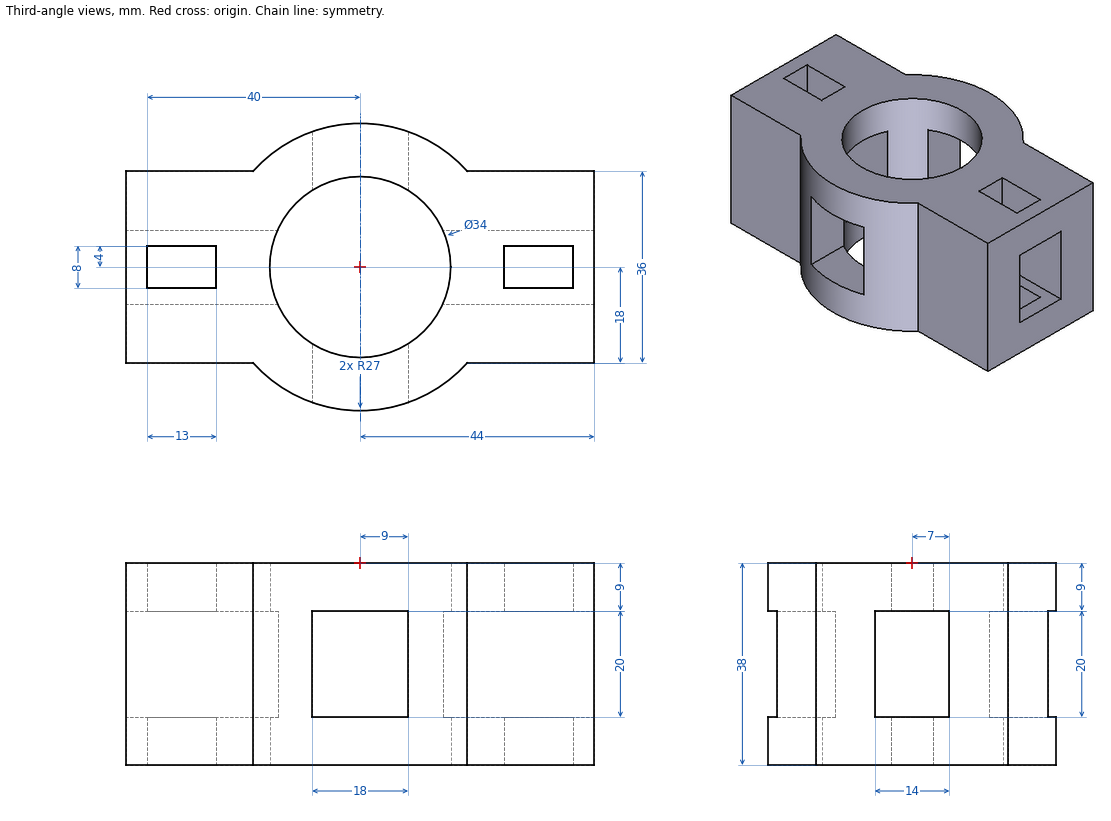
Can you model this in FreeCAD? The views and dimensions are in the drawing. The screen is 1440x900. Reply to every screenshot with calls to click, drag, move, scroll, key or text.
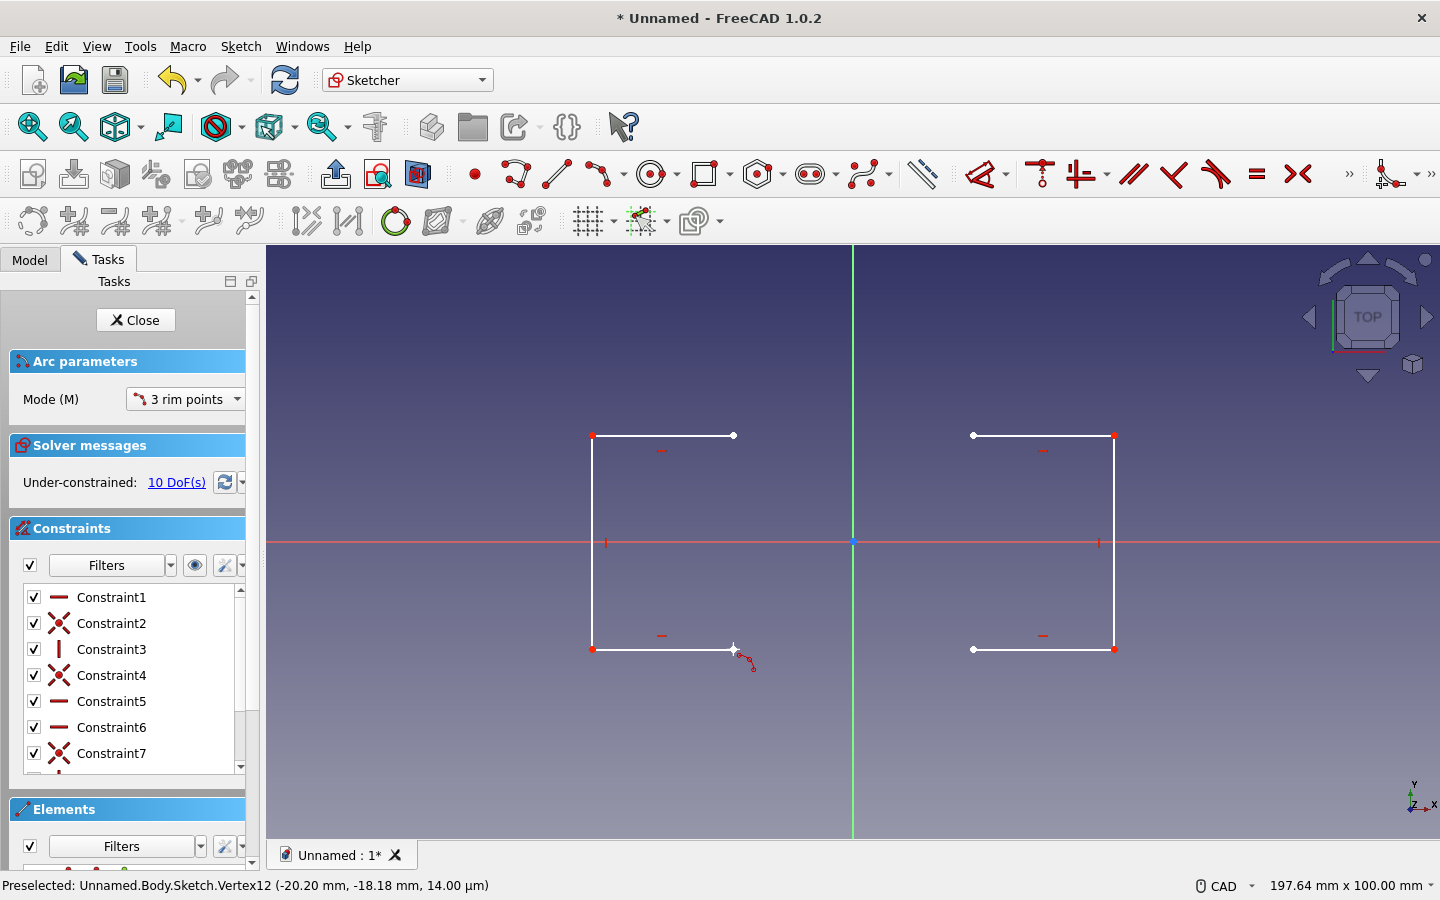
click(973, 436)
click(733, 436)
click(880, 384)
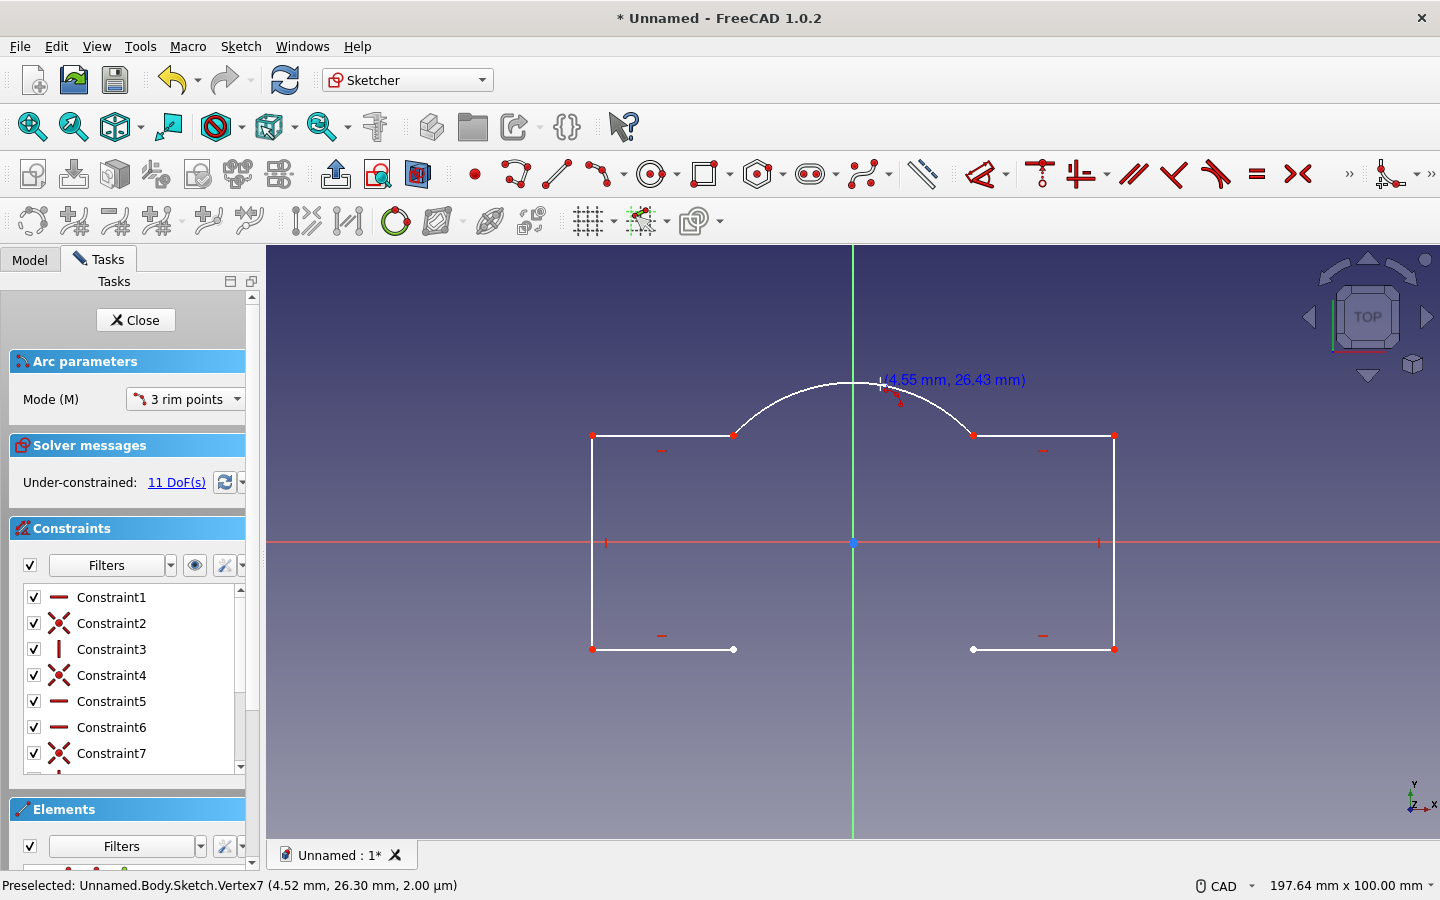
click(733, 650)
click(973, 650)
click(826, 700)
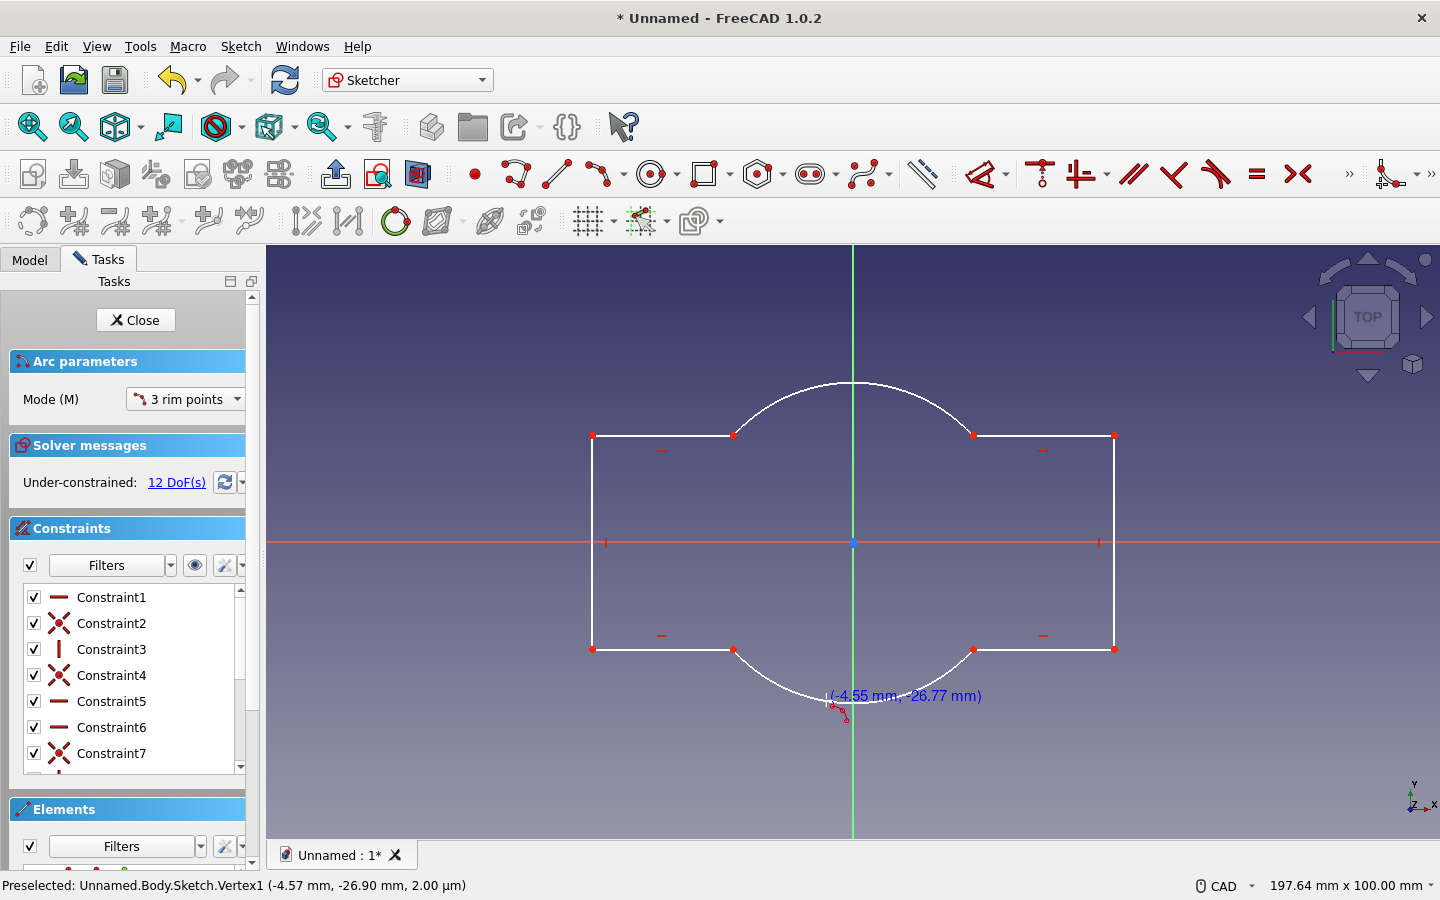
click(704, 174)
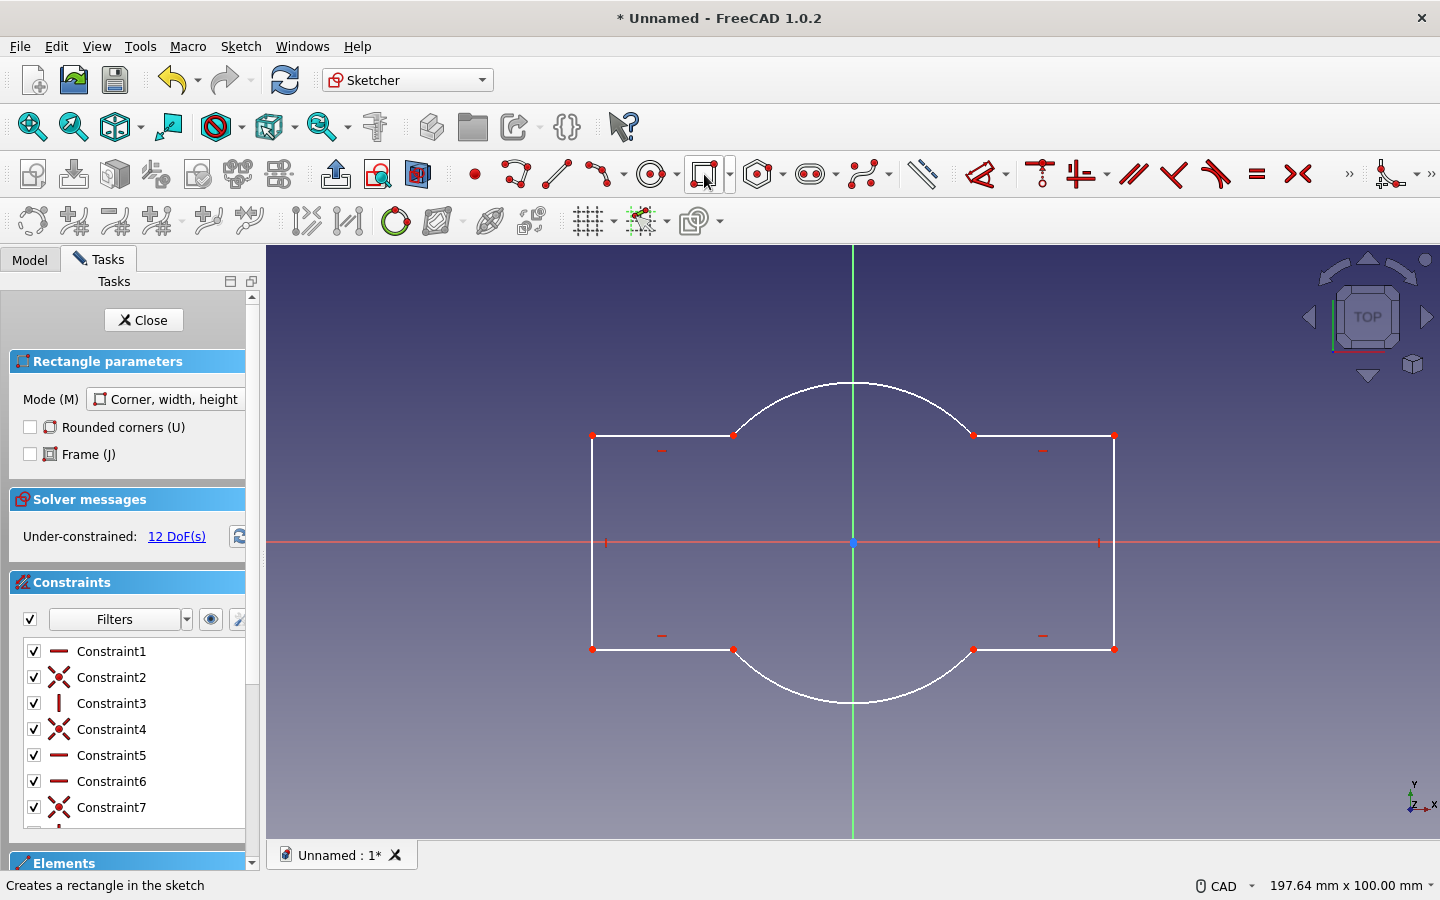
click(615, 518)
click(693, 566)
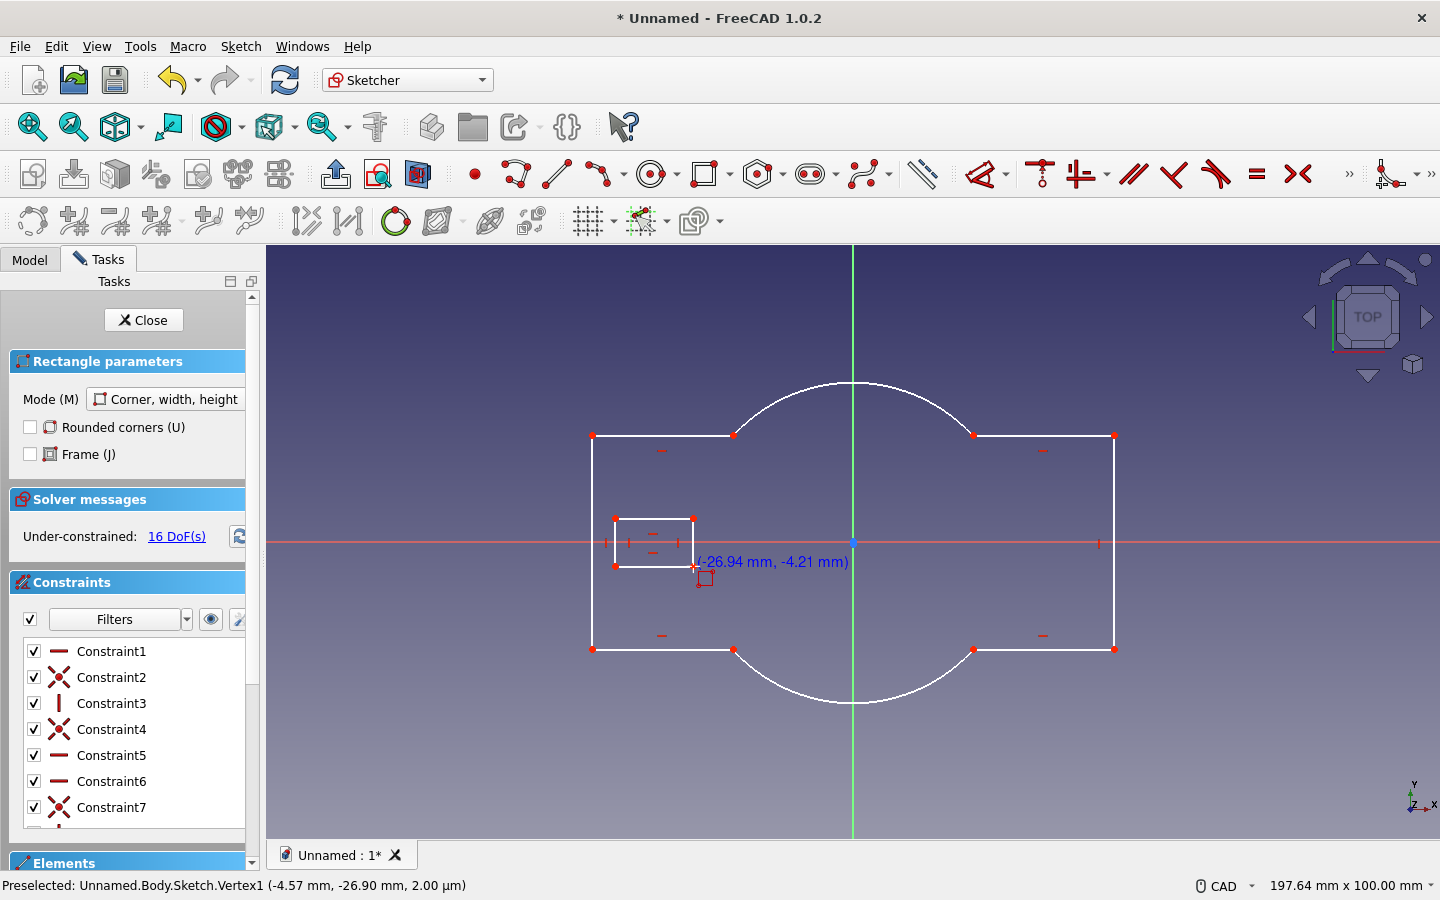
click(1013, 518)
click(1091, 566)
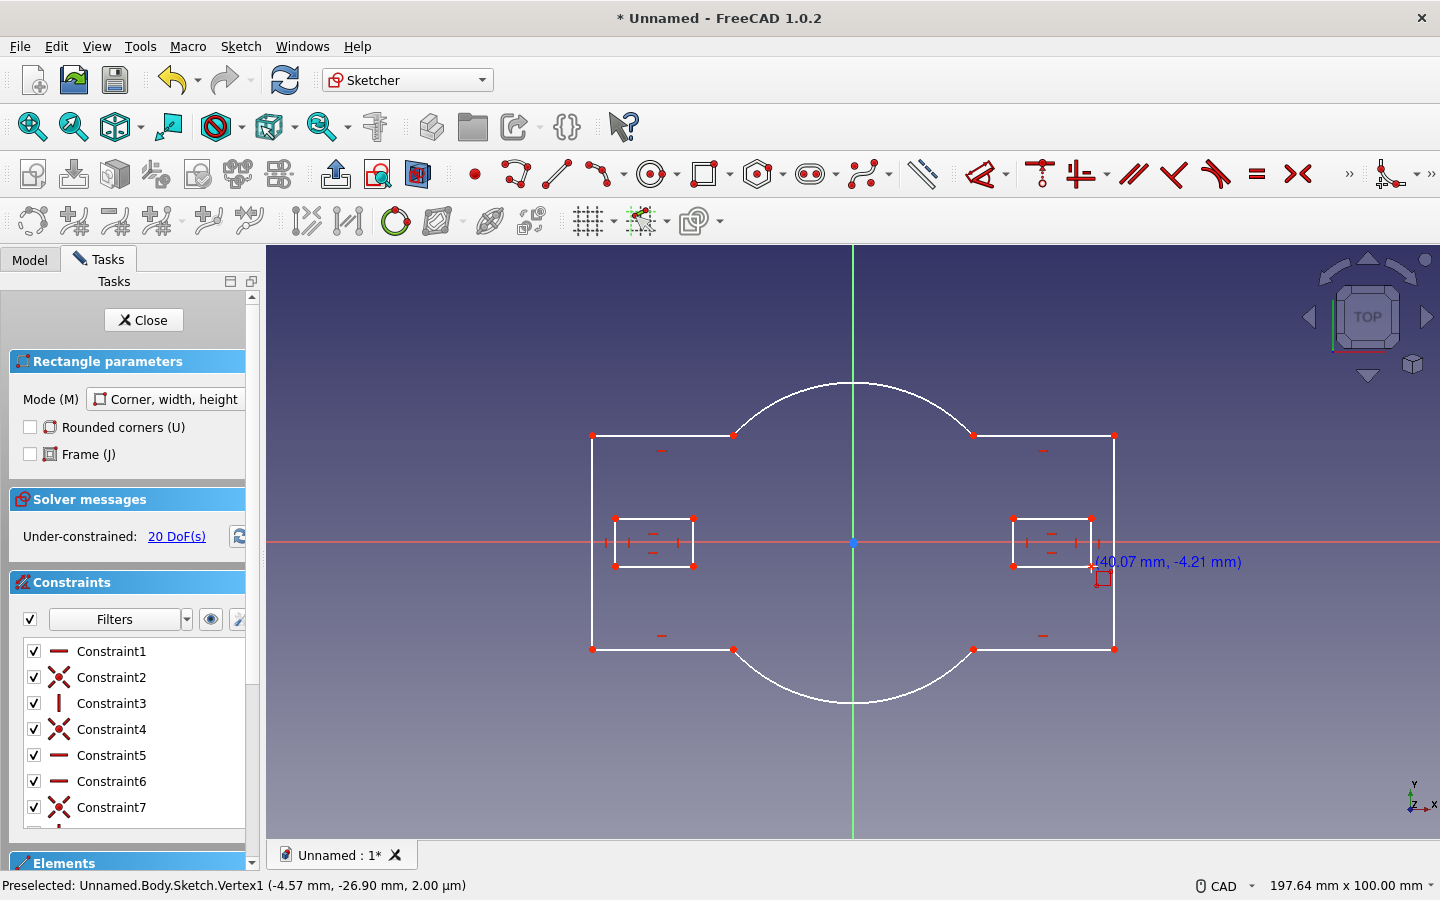
click(650, 174)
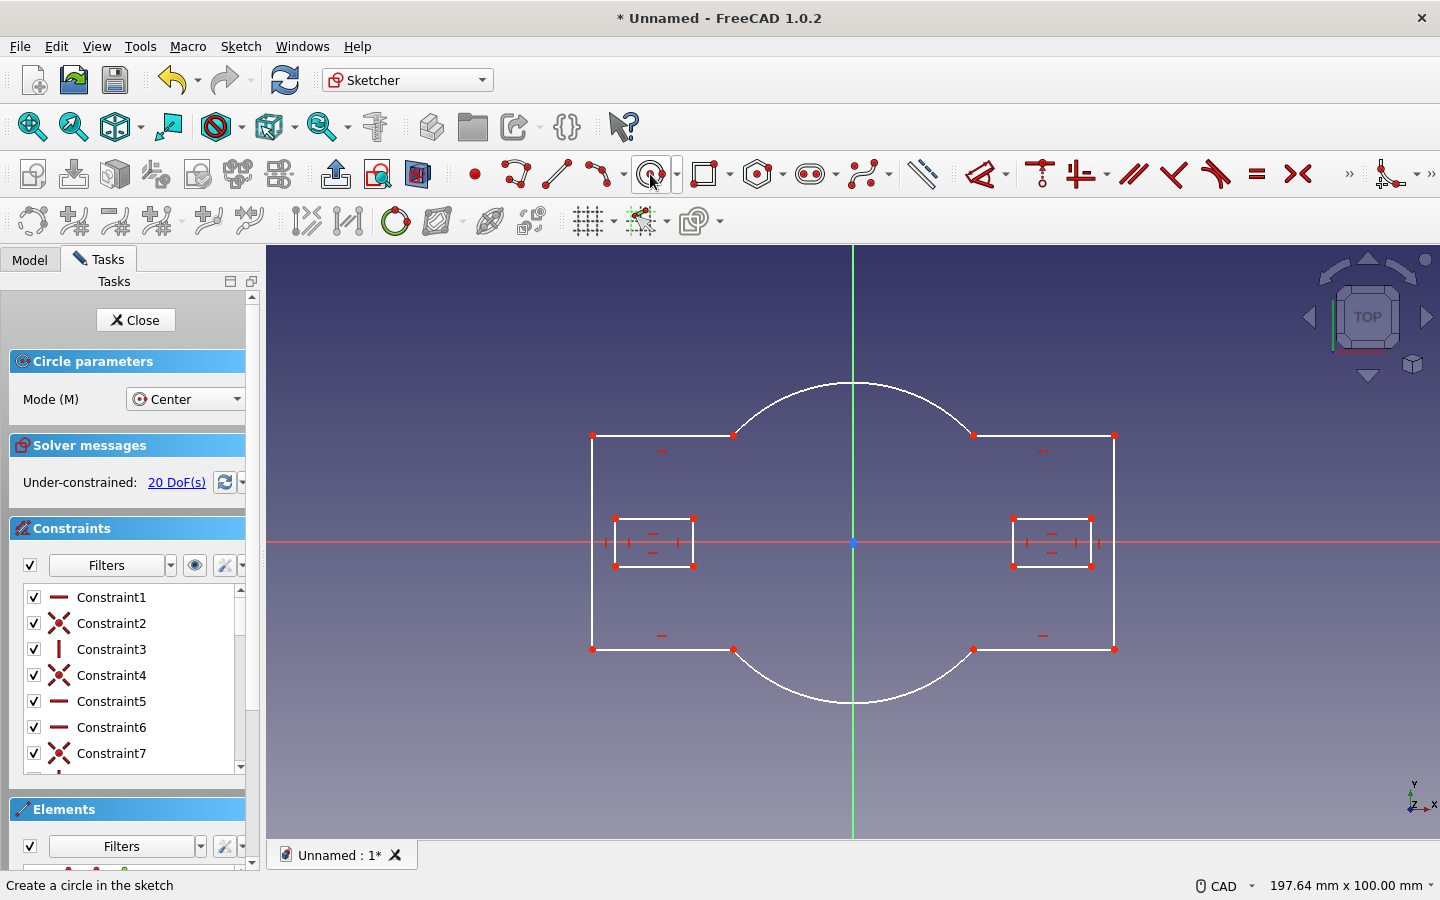
click(853, 542)
click(924, 471)
key(Escape)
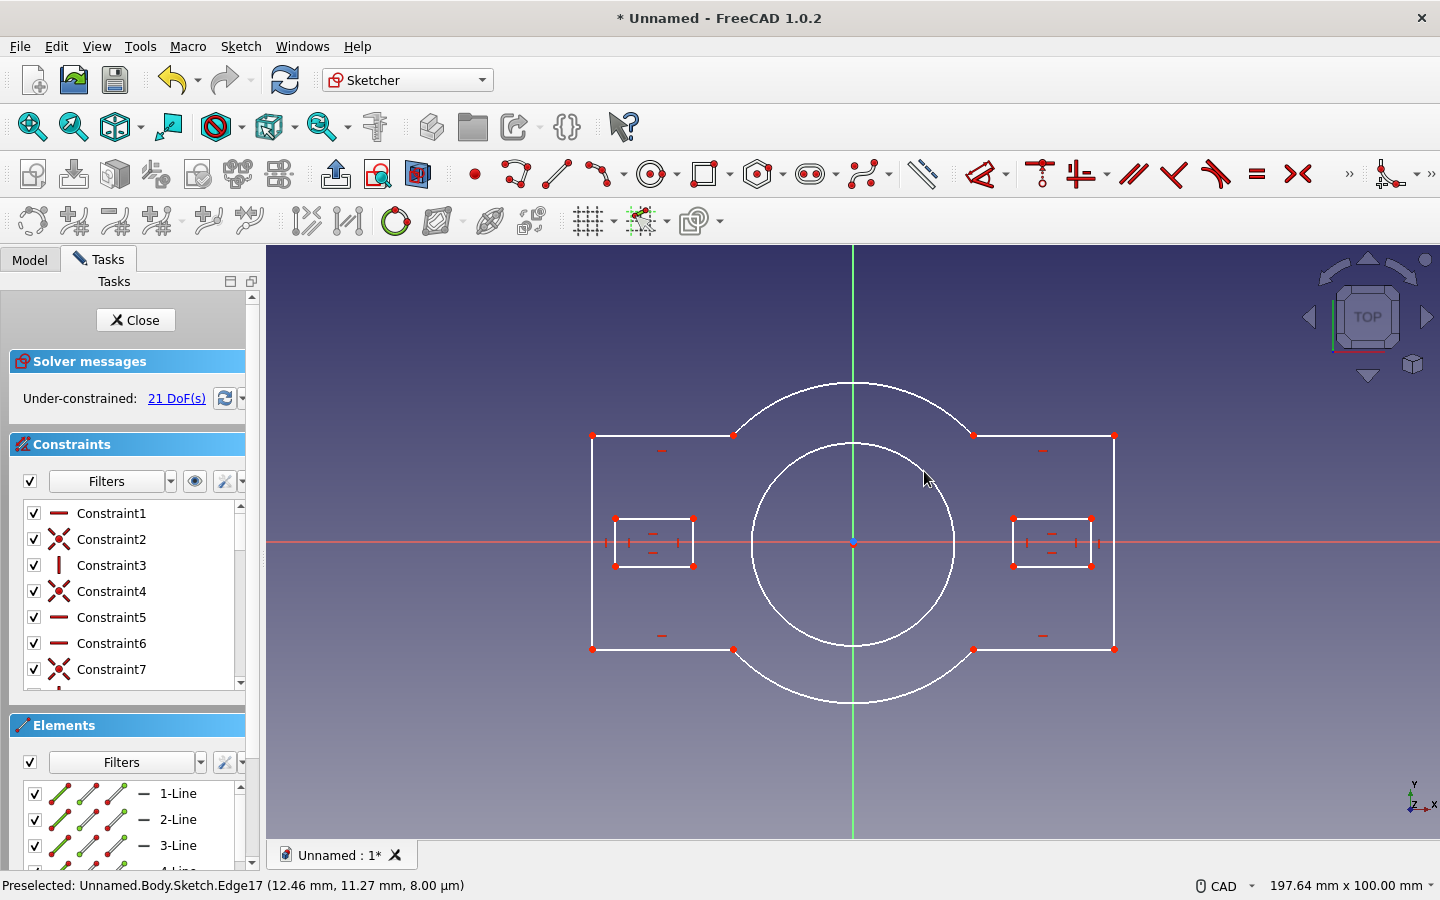
click(925, 473)